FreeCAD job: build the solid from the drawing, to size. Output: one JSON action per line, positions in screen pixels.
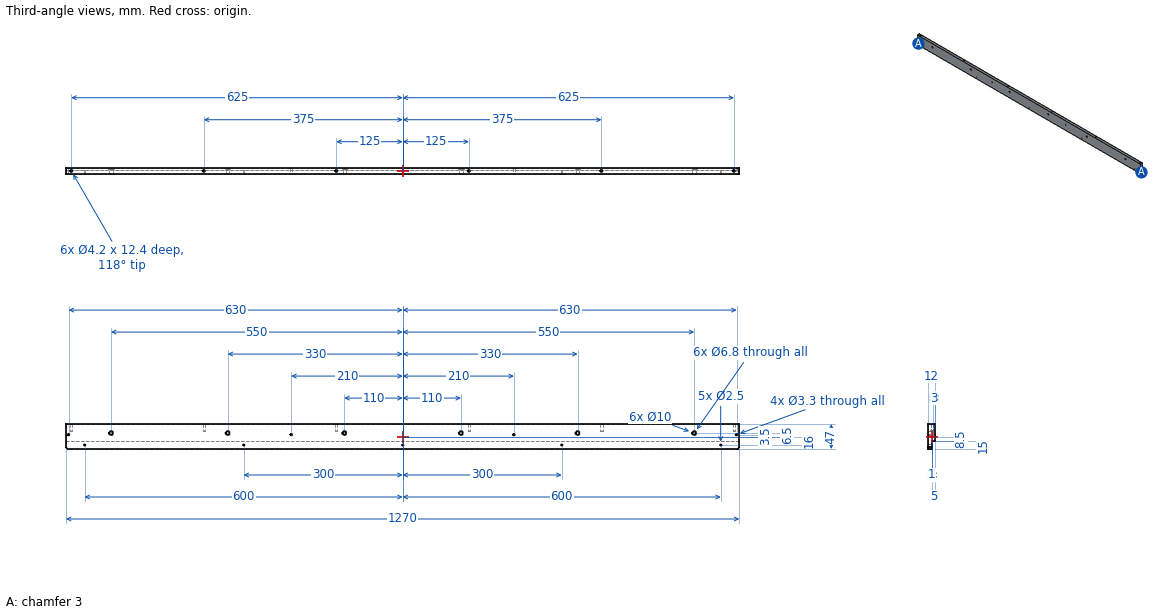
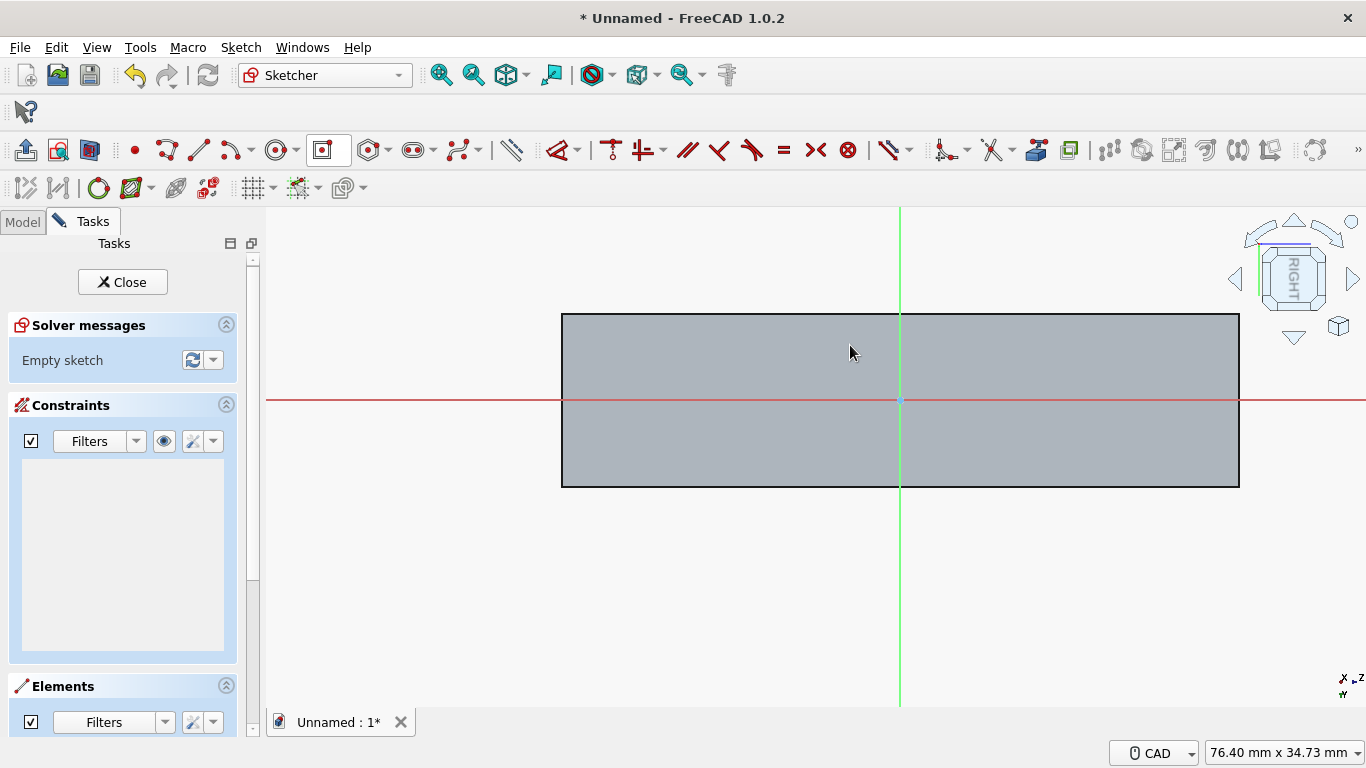
{"action": "scroll", "coordinate": [711, 427], "scroll_direction": "up", "scroll_amount": 3}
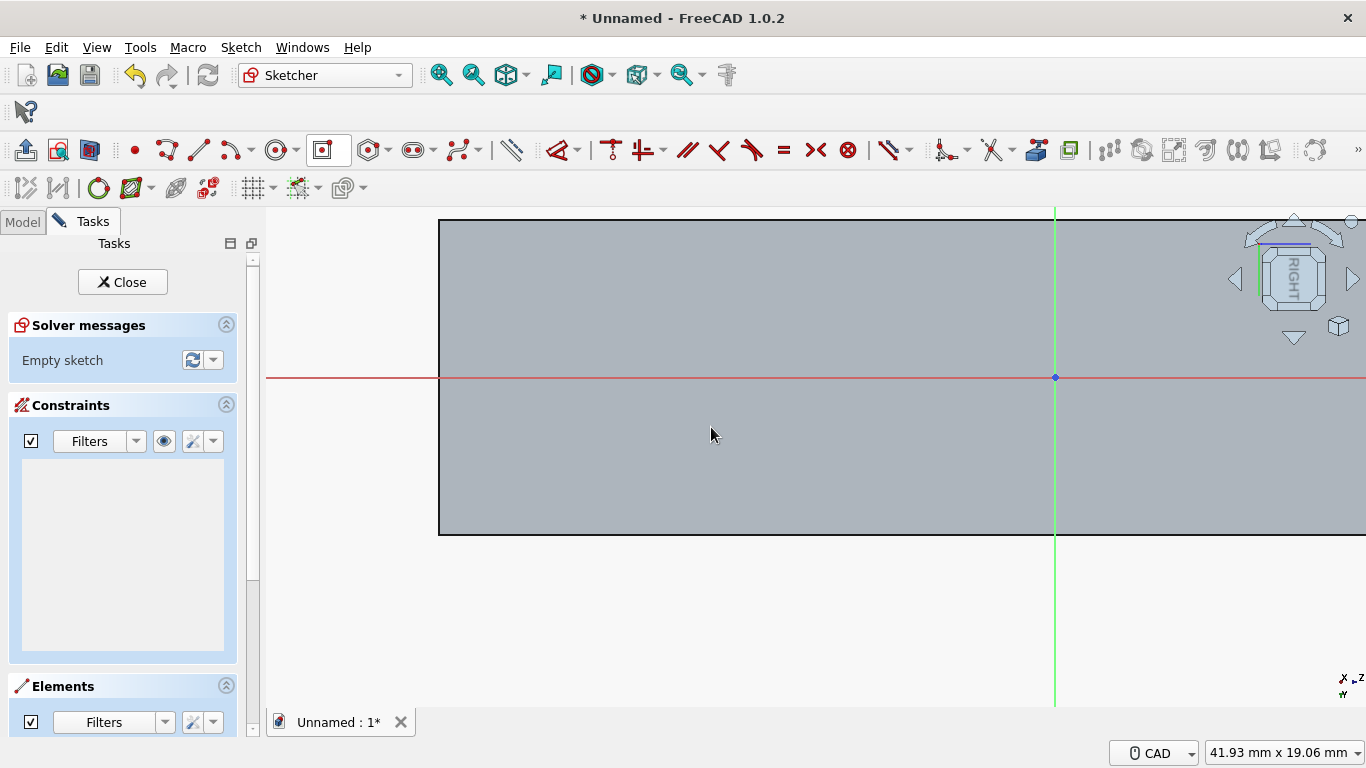
{"action": "key", "text": "g r"}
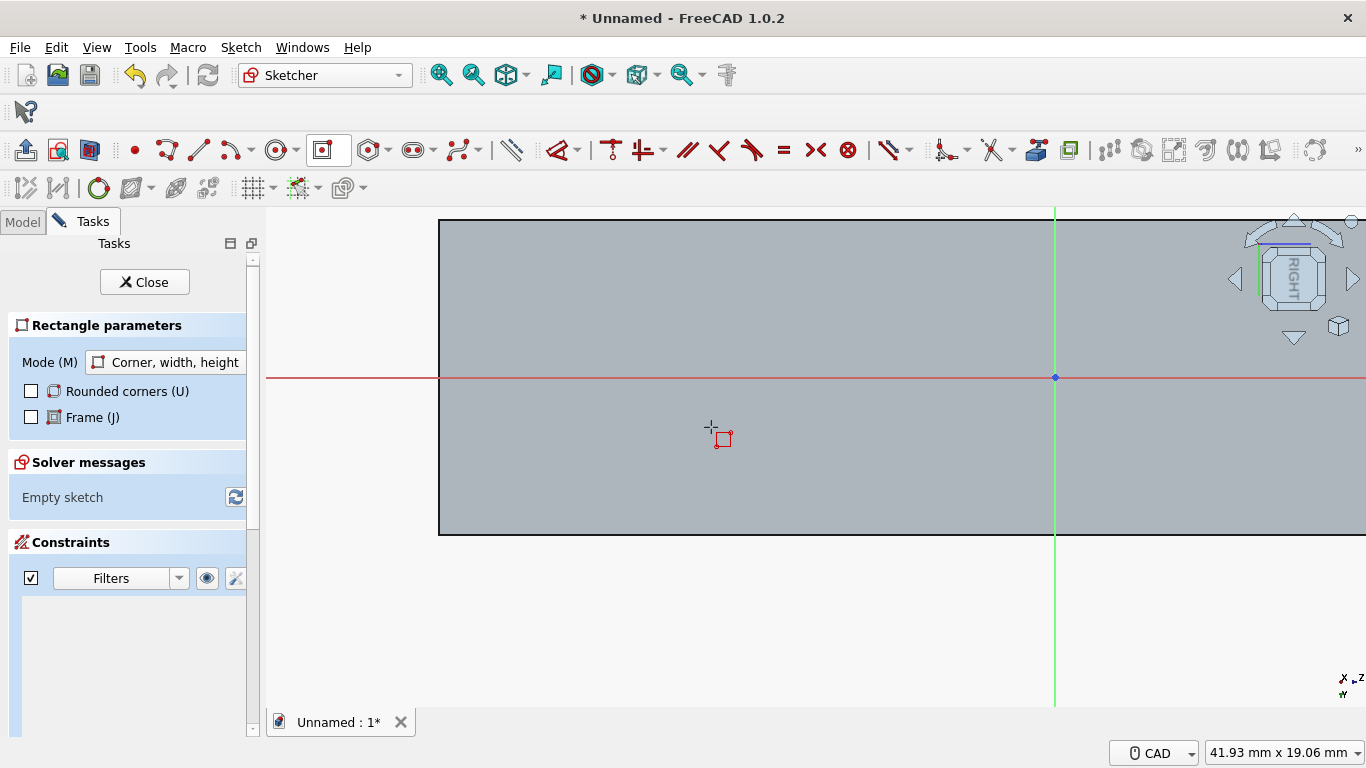
{"action": "left_click", "coordinate": [439, 404]}
{"action": "mouse_move", "coordinate": [832, 535]}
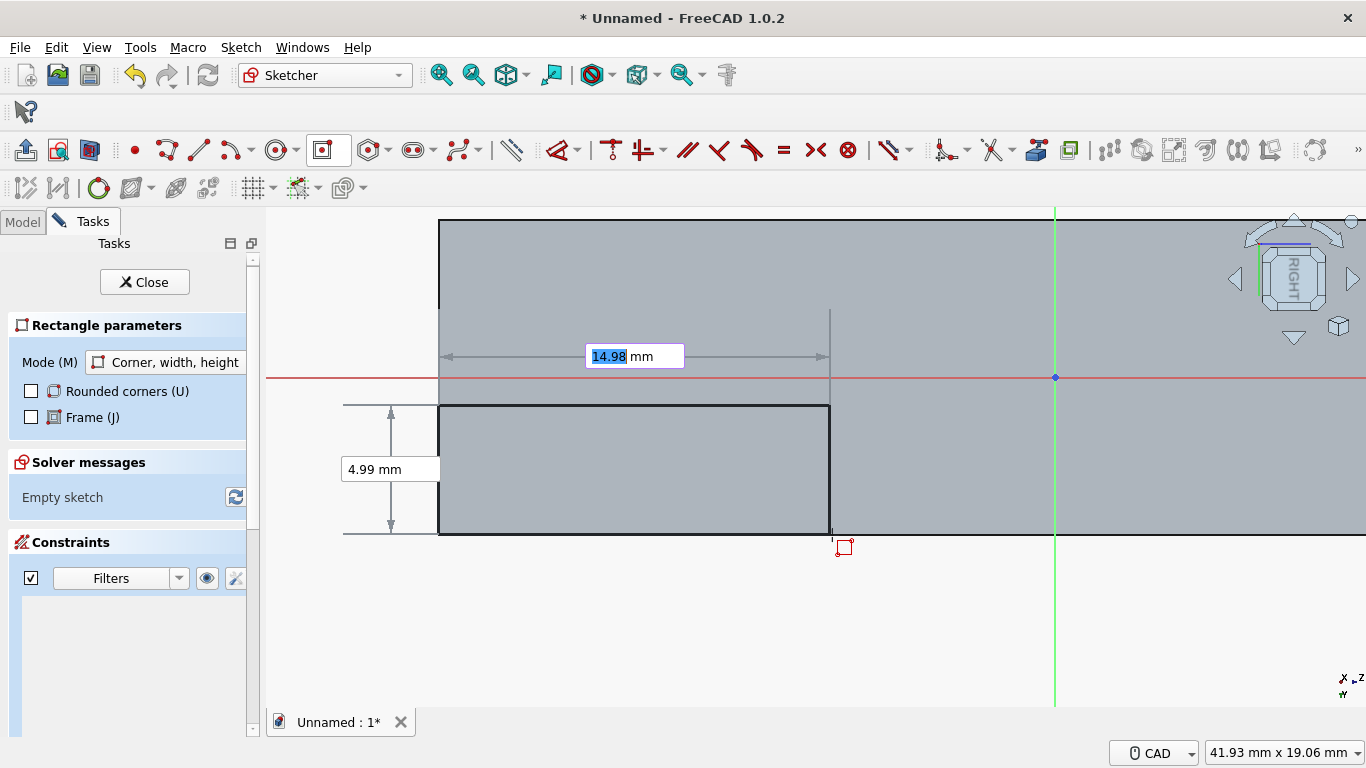
{"action": "type", "text": "15"}
{"action": "key", "text": "Tab"}
{"action": "type", "text": "5"}
{"action": "key", "text": "Return"}
{"action": "key", "text": "Escape"}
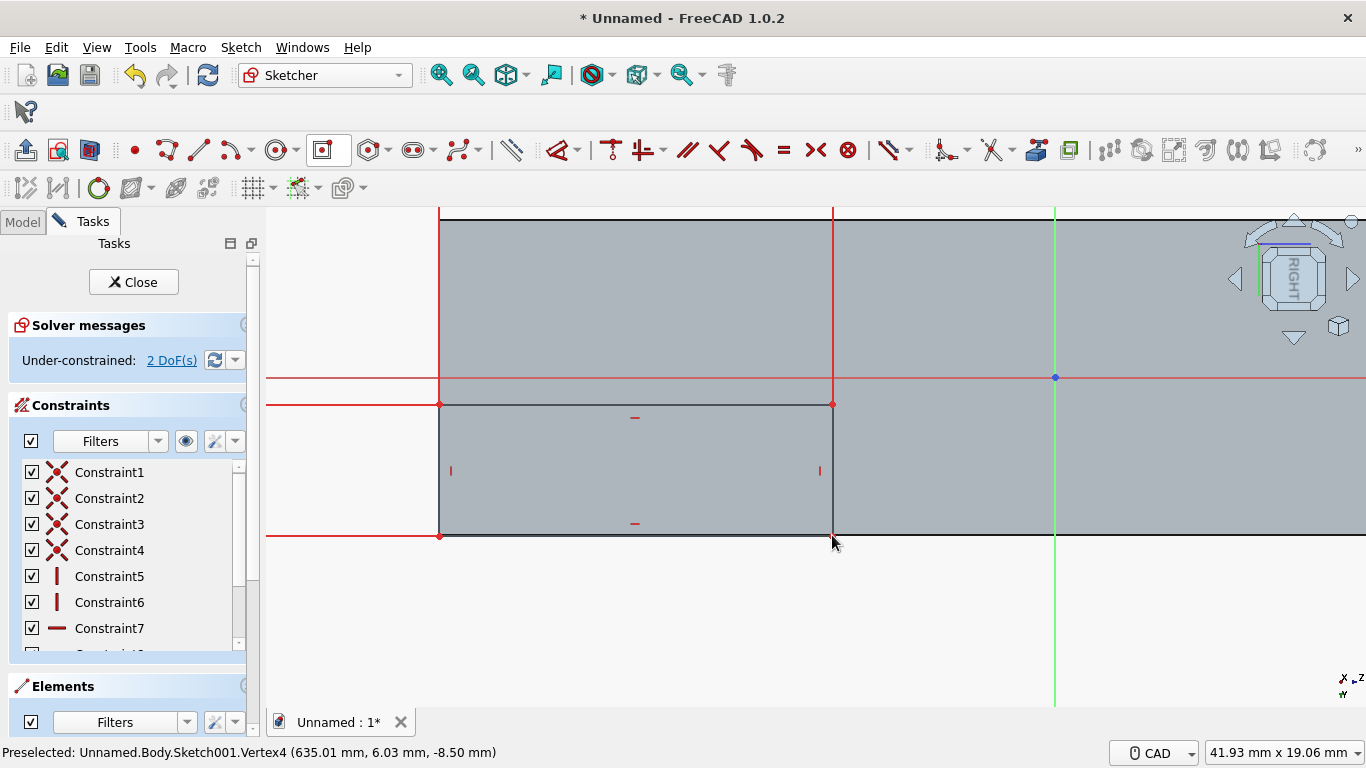
{"action": "left_click", "coordinate": [558, 150]}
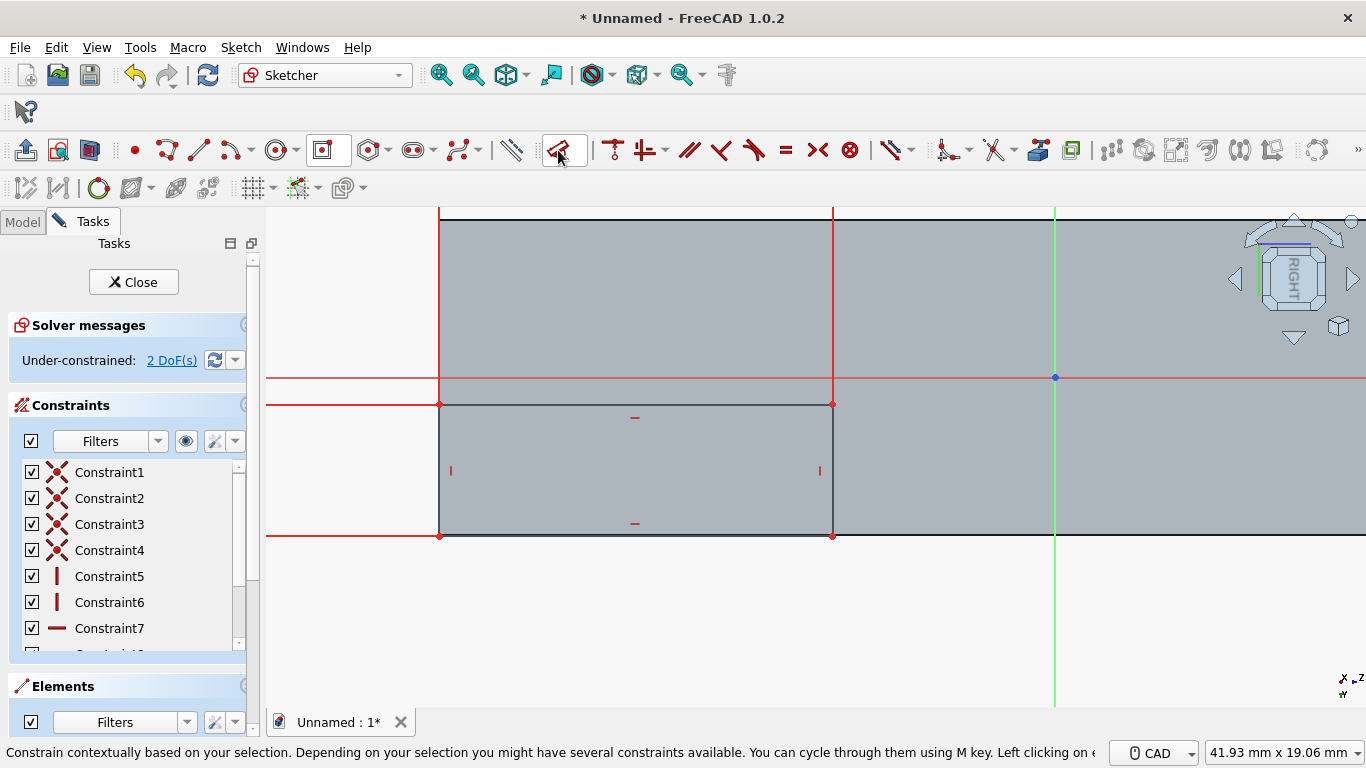
{"action": "scroll", "coordinate": [439, 405], "scroll_direction": "up", "scroll_amount": 3}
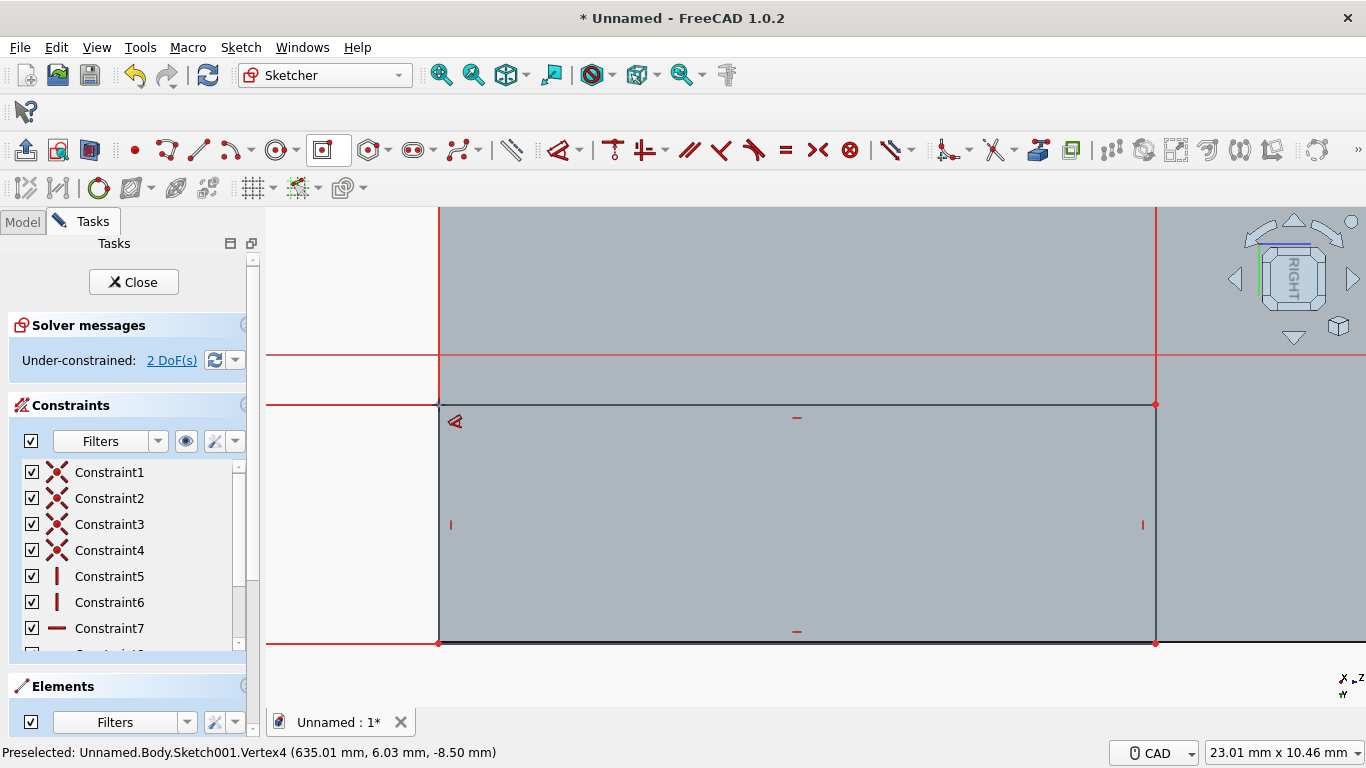
{"action": "left_click", "coordinate": [439, 405]}
{"action": "left_click", "coordinate": [405, 380]}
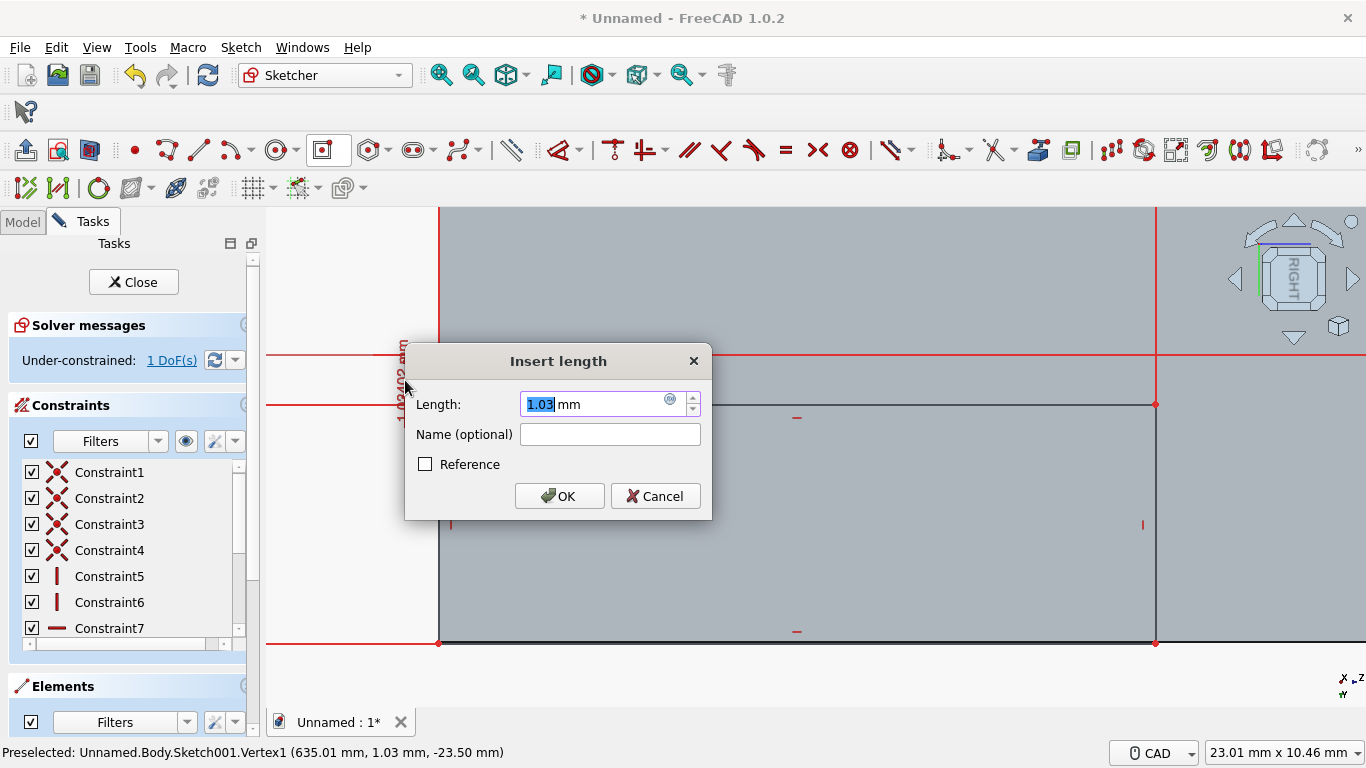
{"action": "type", "text": "1"}
{"action": "key", "text": "Return"}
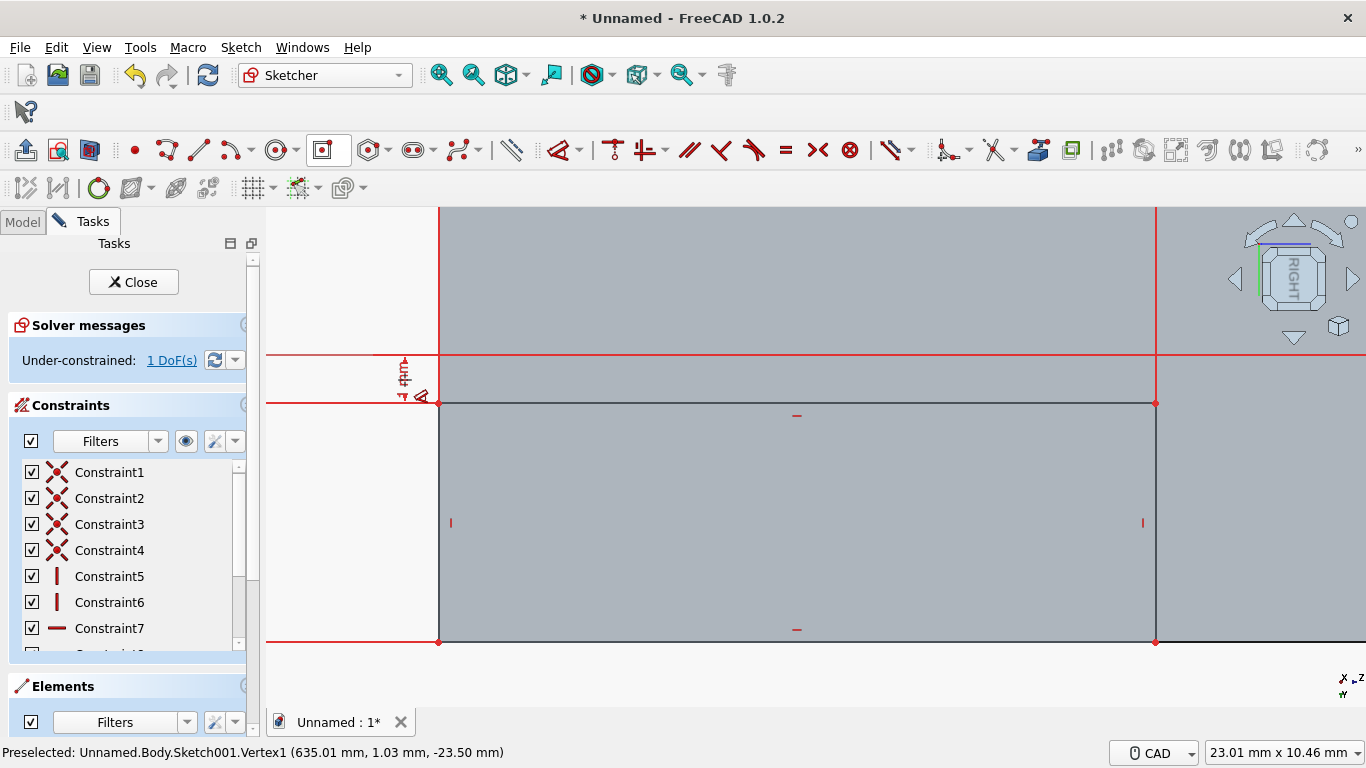
{"action": "left_click", "coordinate": [1156, 642]}
{"action": "left_click", "coordinate": [1178, 321]}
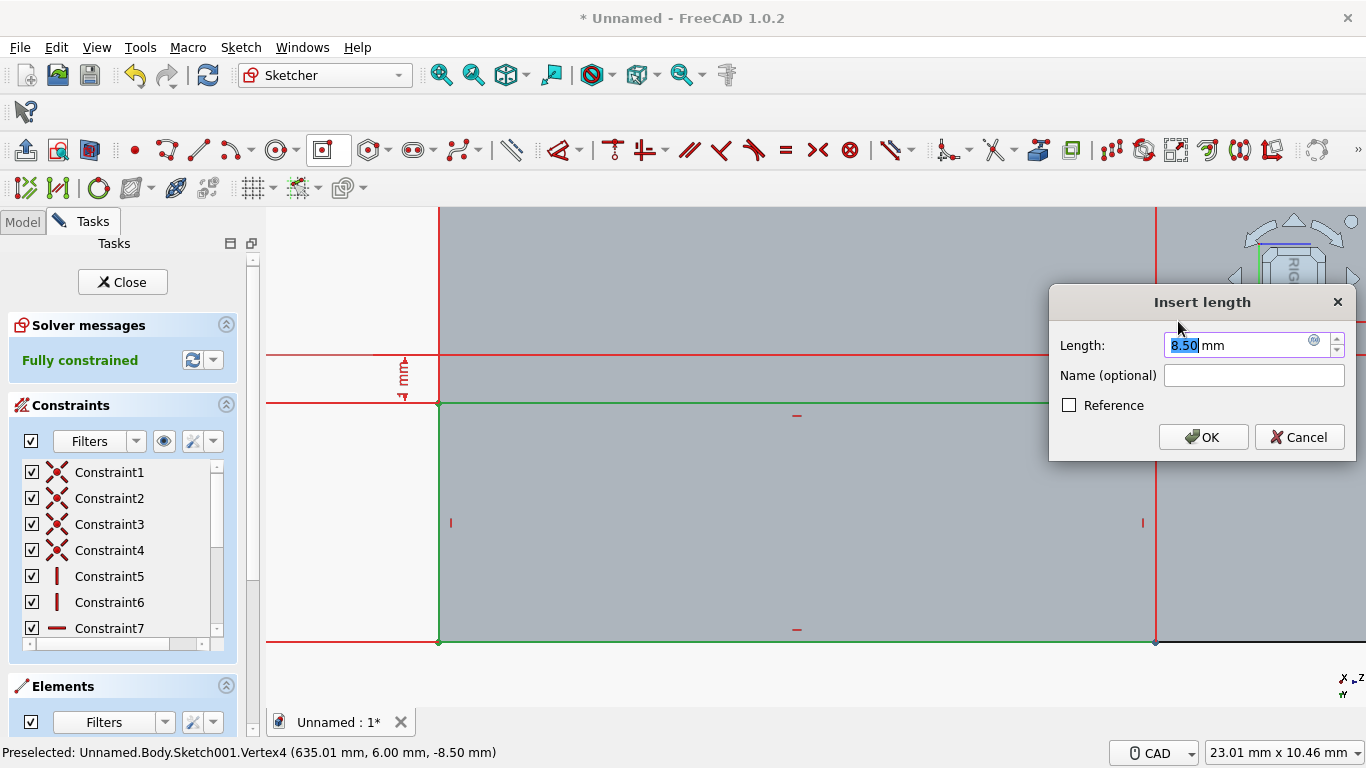
{"action": "type", "text": "8.5"}
{"action": "key", "text": "Return"}
{"action": "key", "text": "Escape"}